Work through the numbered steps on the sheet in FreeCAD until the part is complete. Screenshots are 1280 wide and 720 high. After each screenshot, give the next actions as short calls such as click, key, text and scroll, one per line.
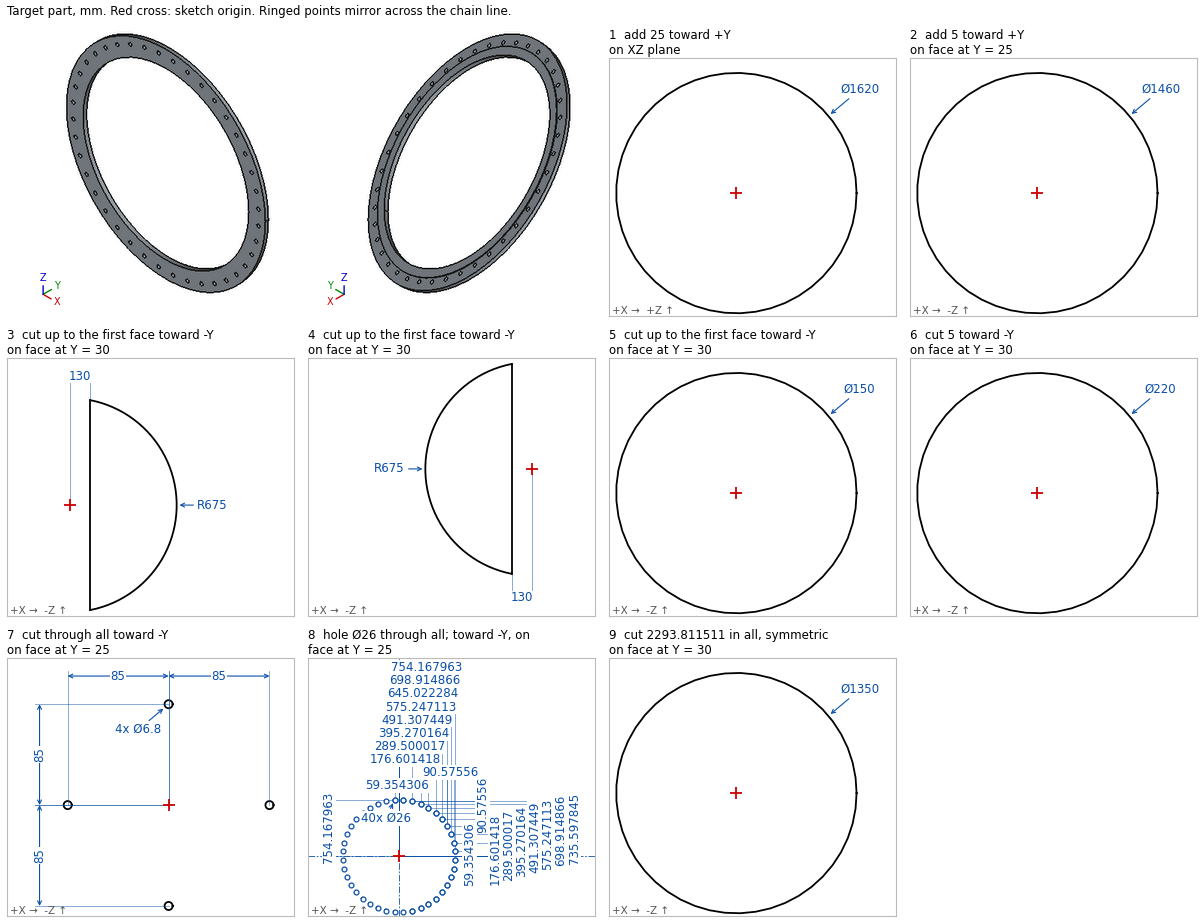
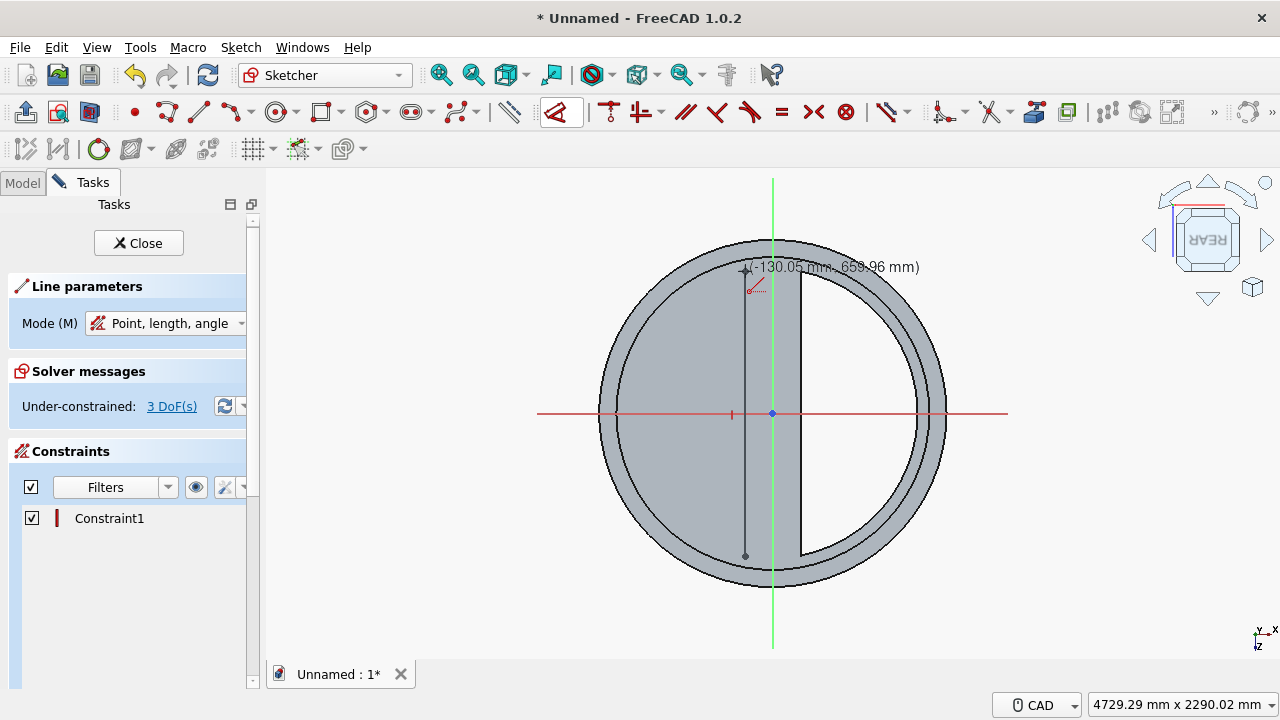
key(g)
key(3)
key(a)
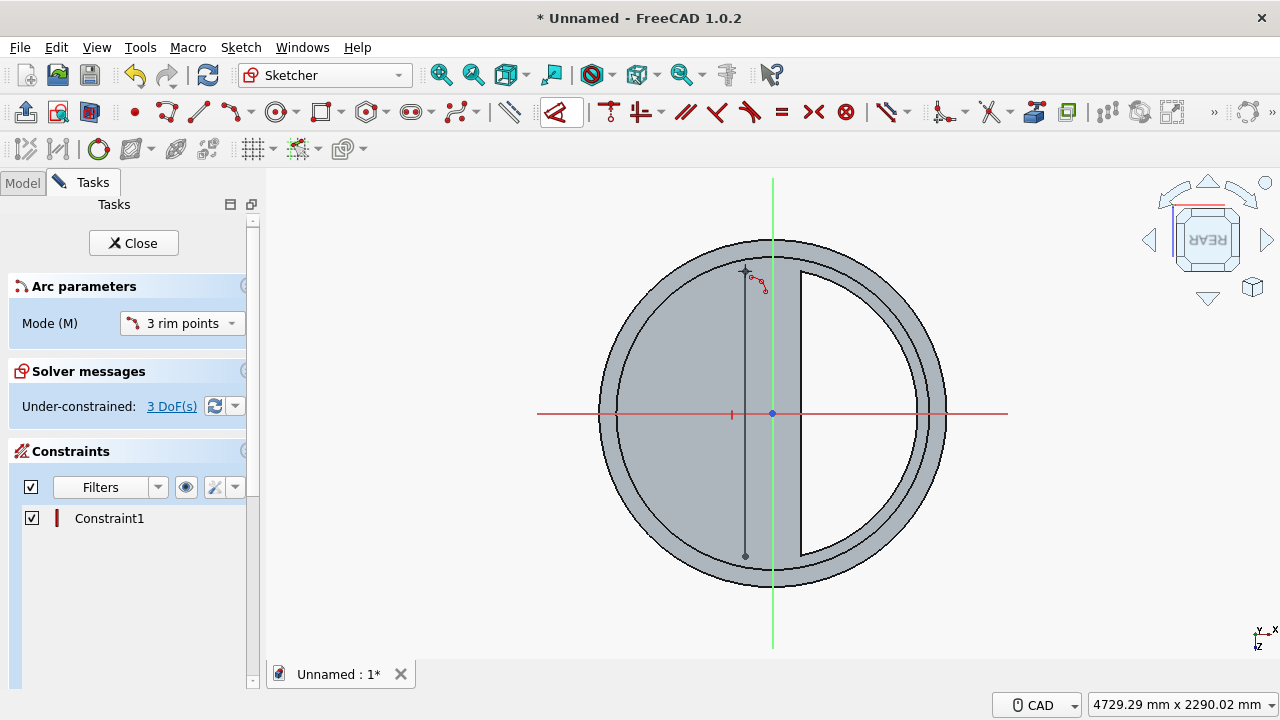
click(745, 272)
click(745, 557)
click(634, 374)
key(Escape)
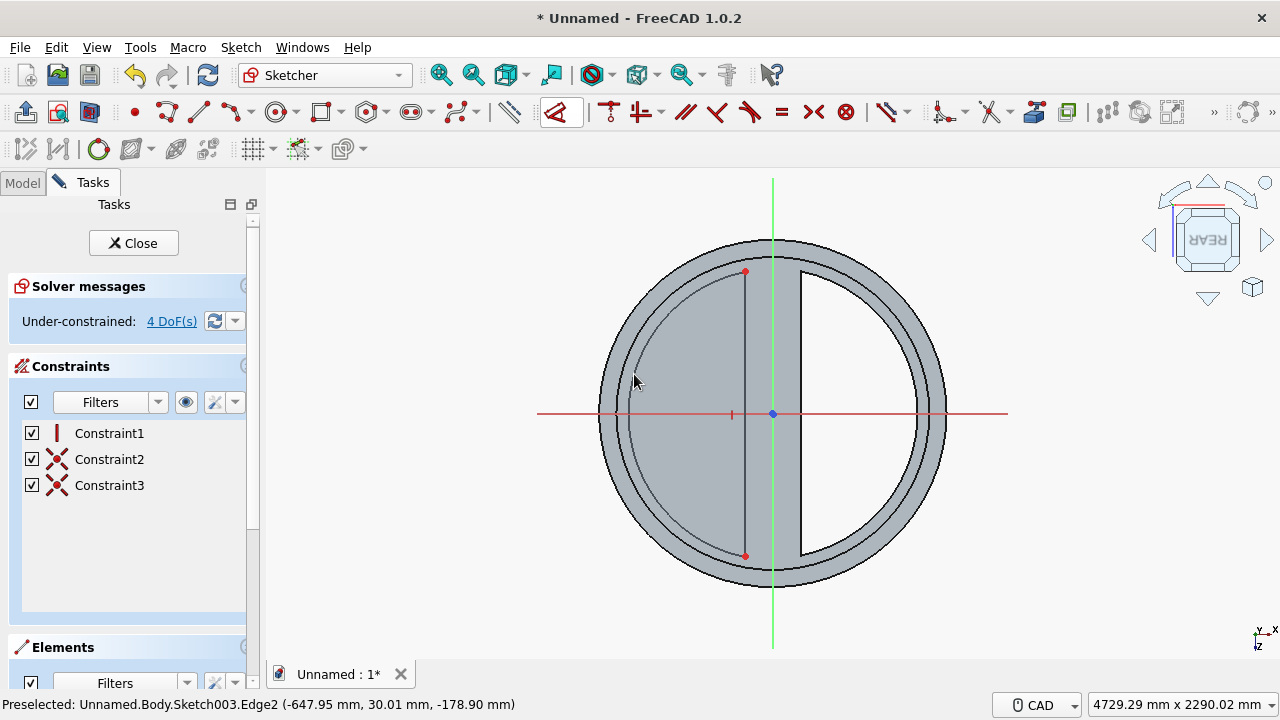
drag(763, 403, 784, 425)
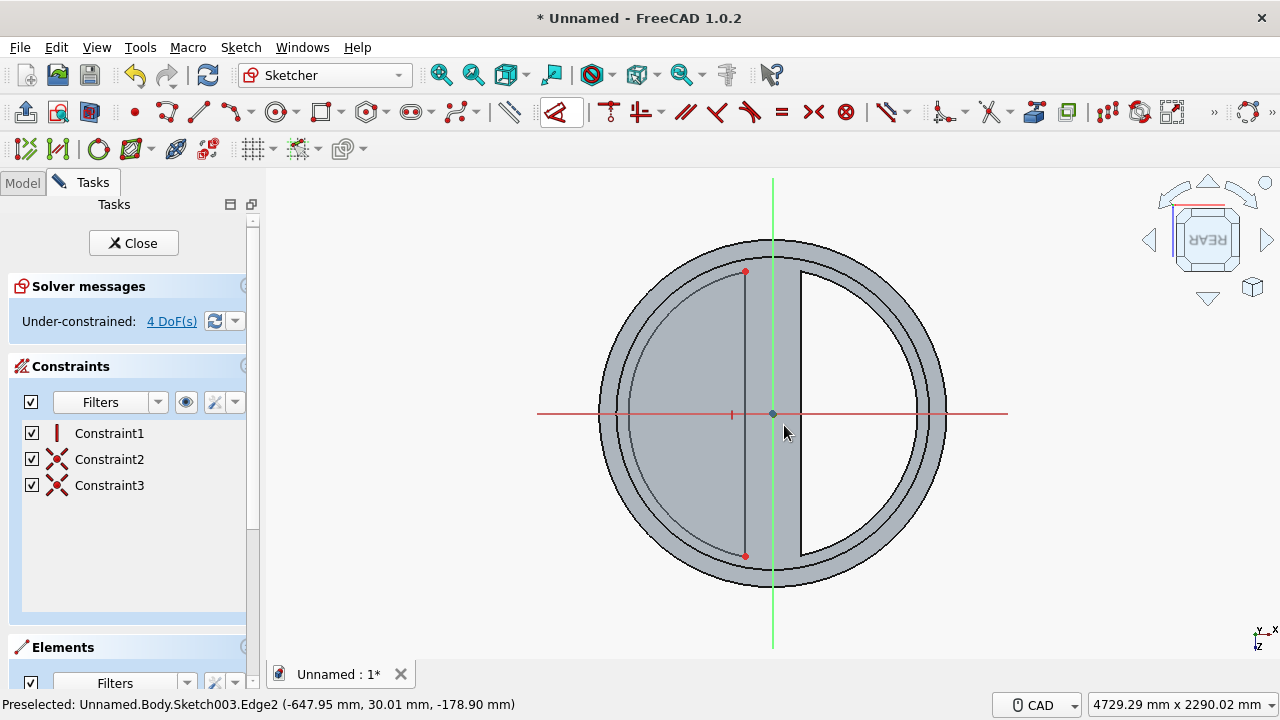
key(c)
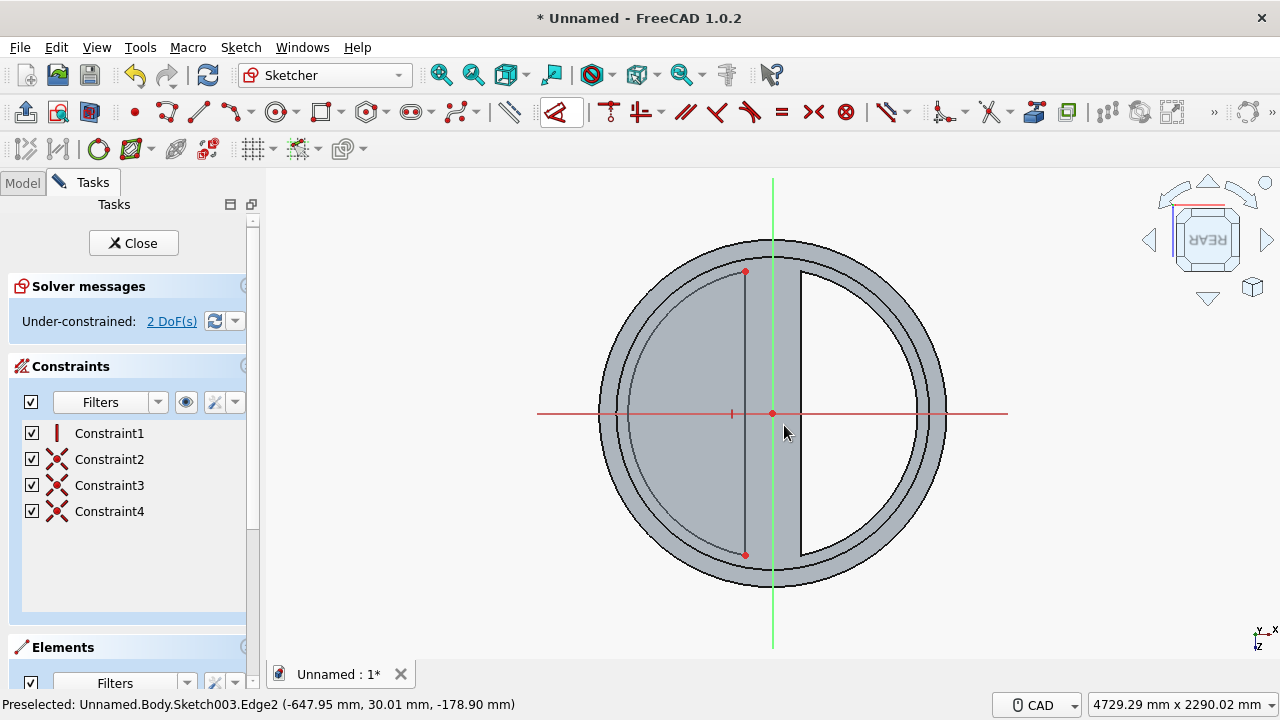
click(650, 338)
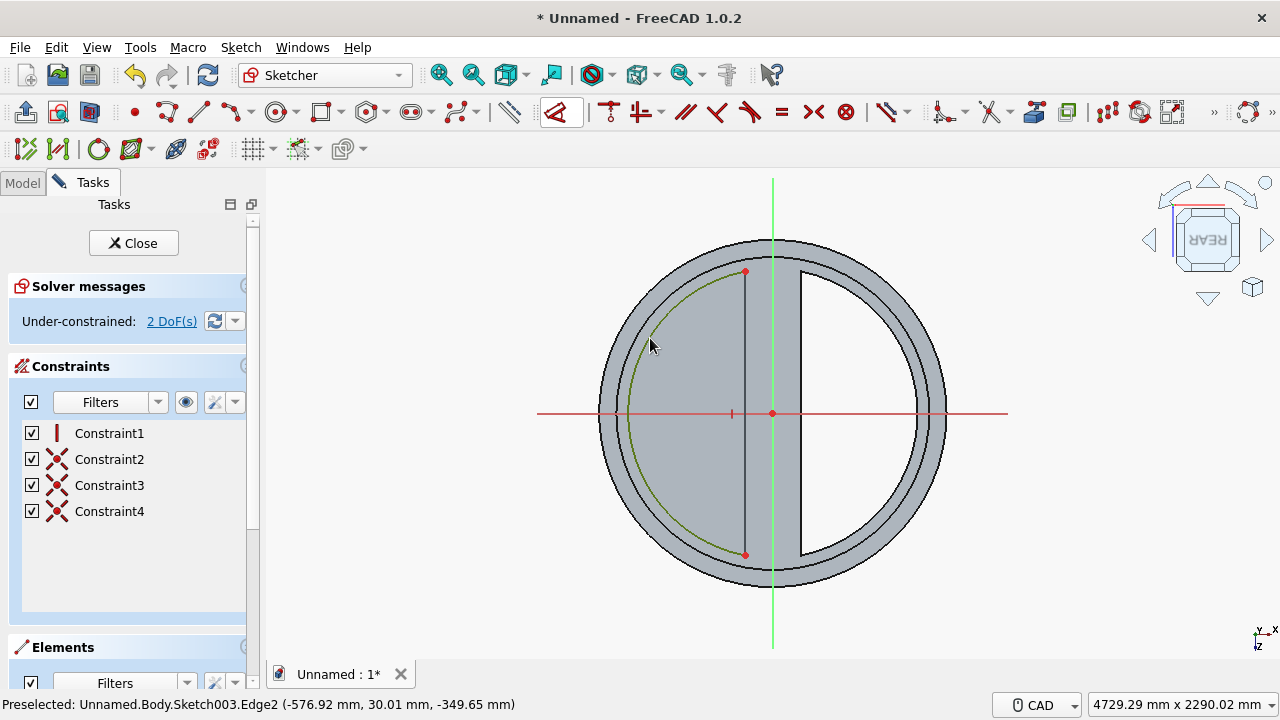
click(578, 112)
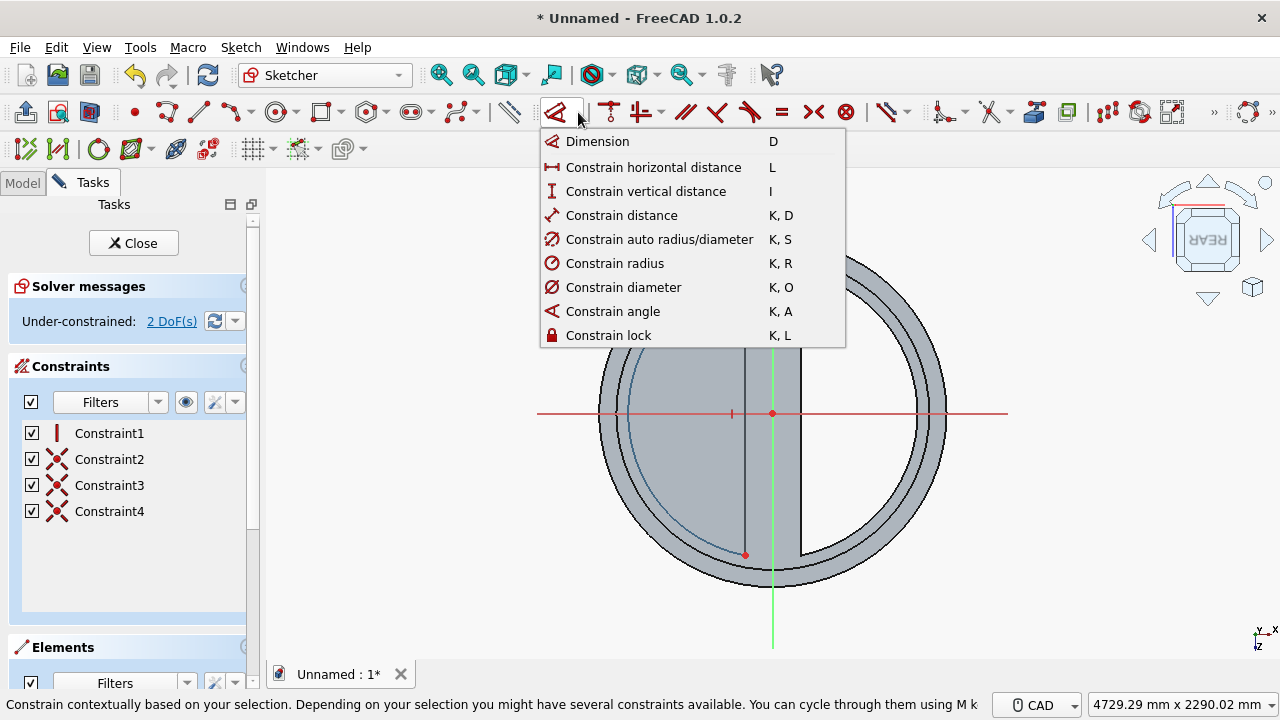
click(693, 263)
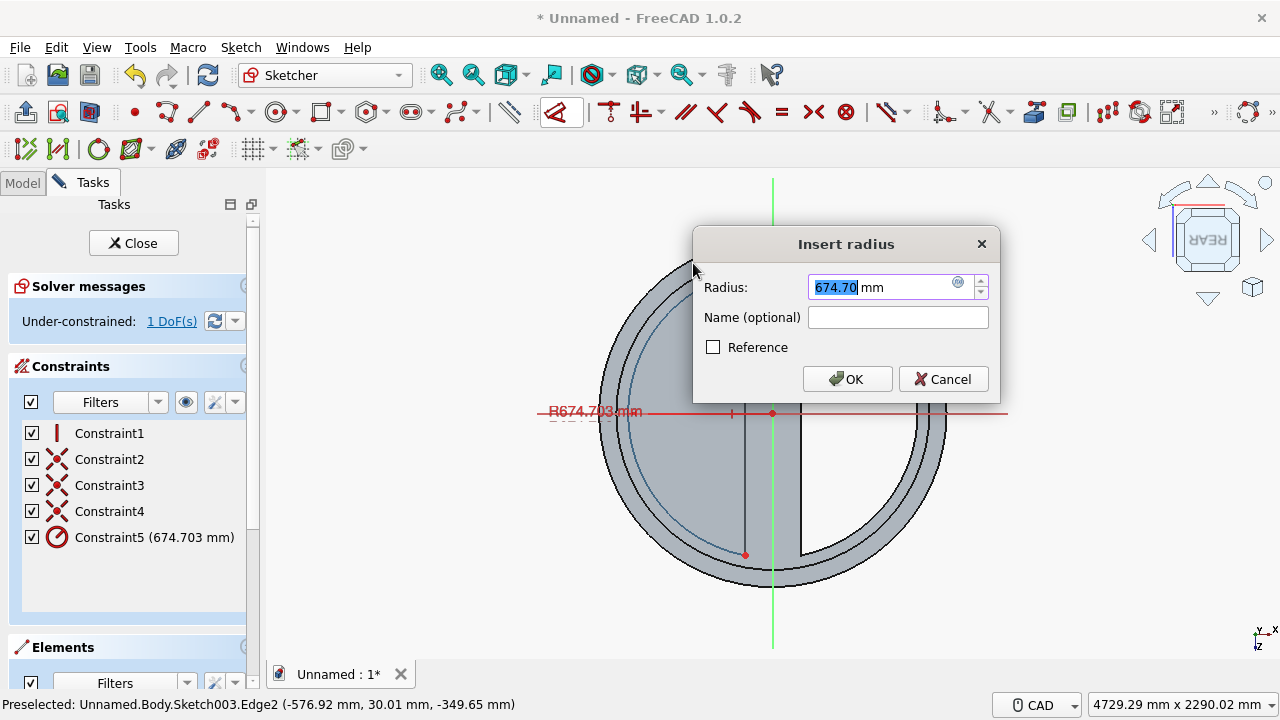
text(675)
key(Return)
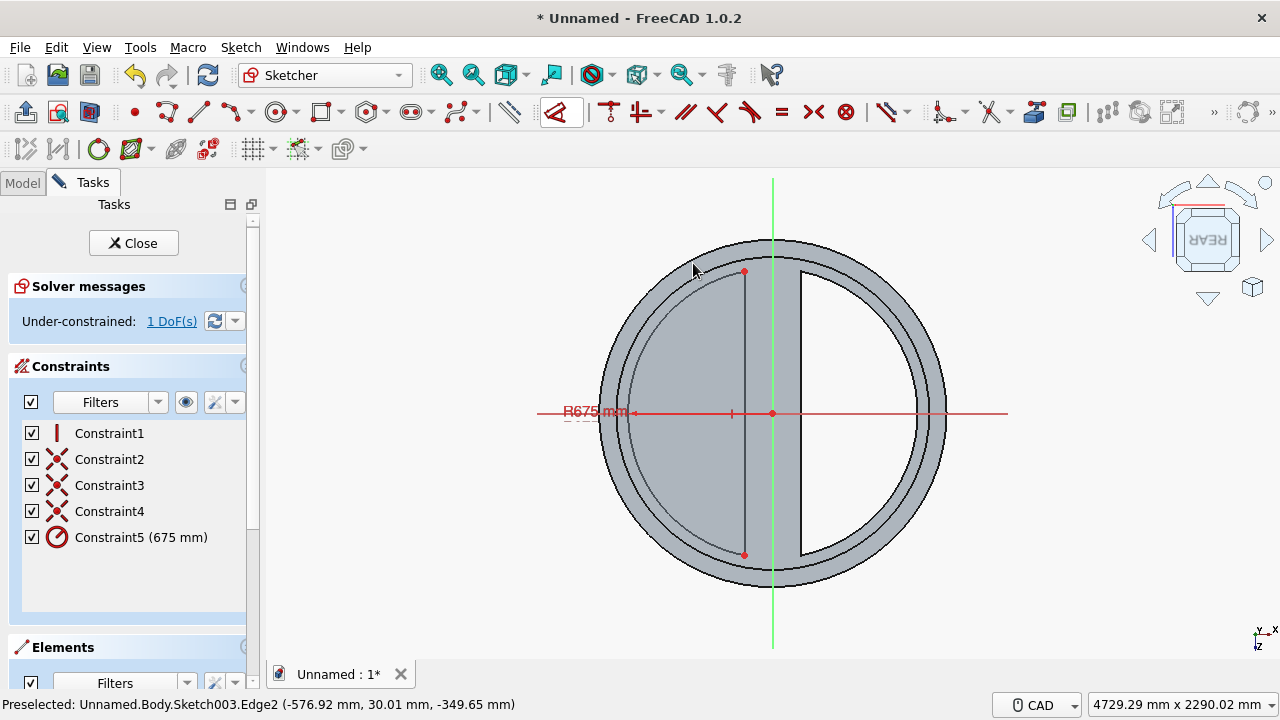
scroll(745, 556, up, 2)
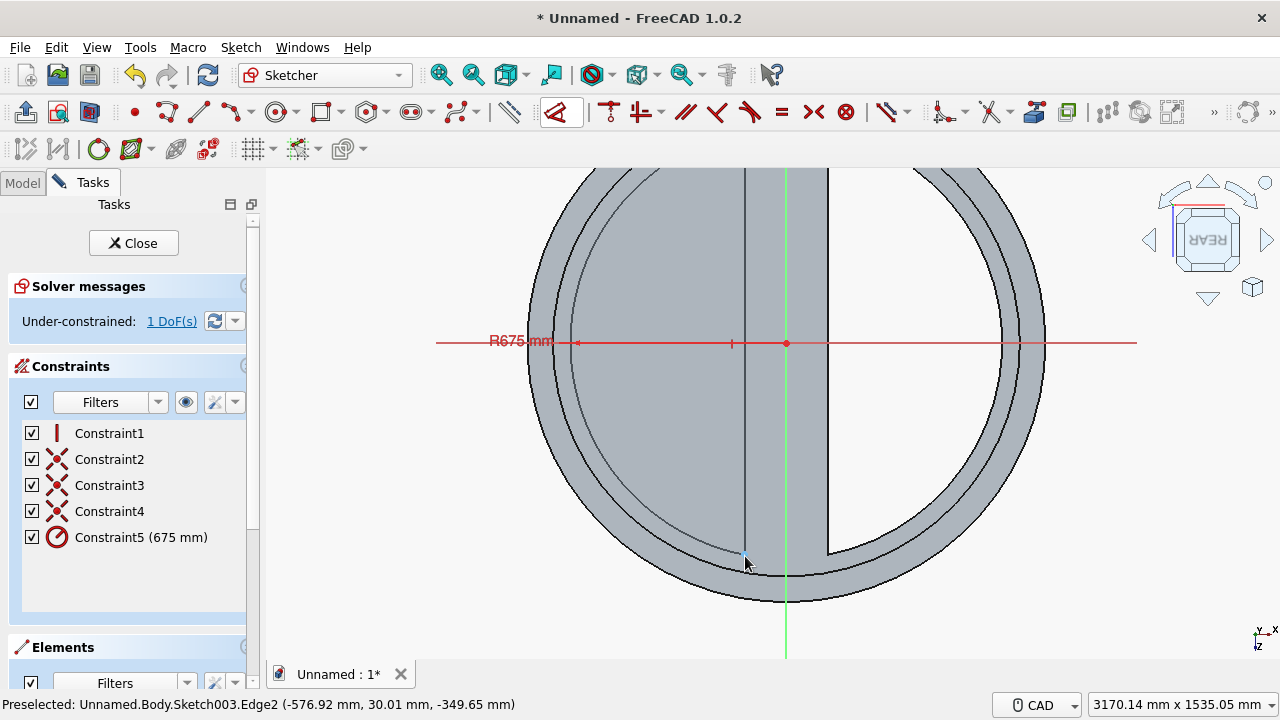
click(745, 555)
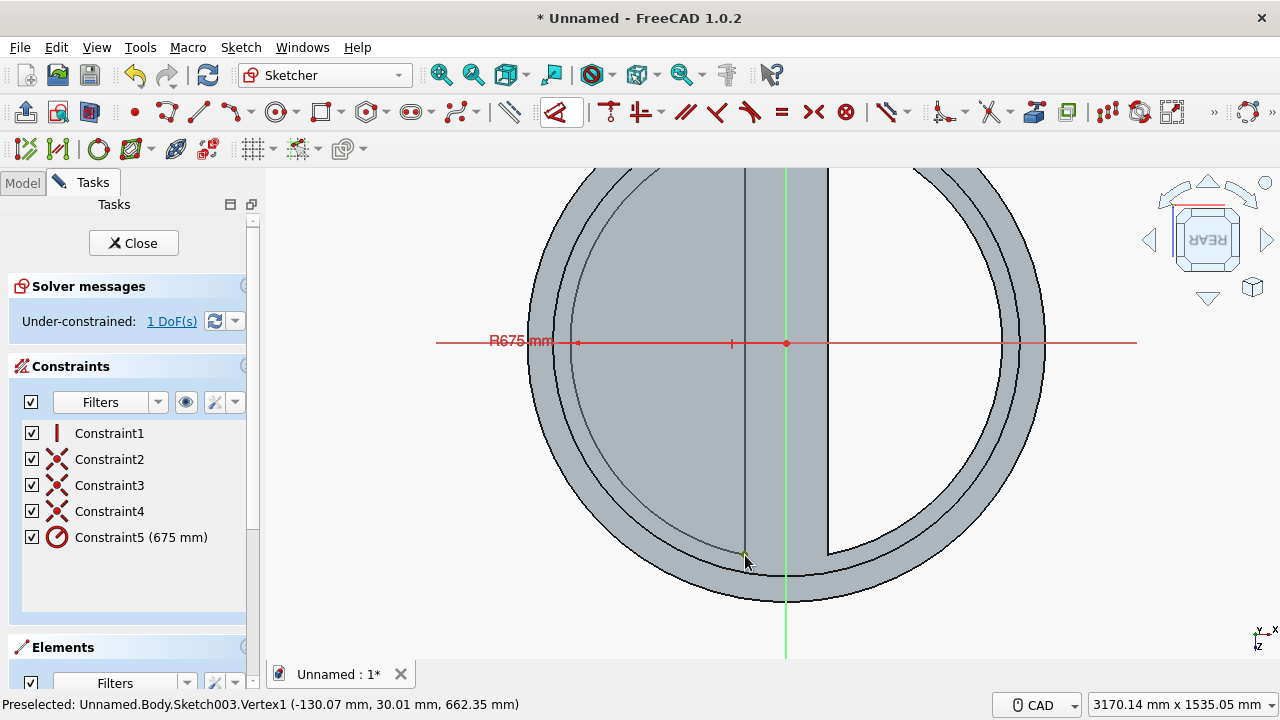
key(l)